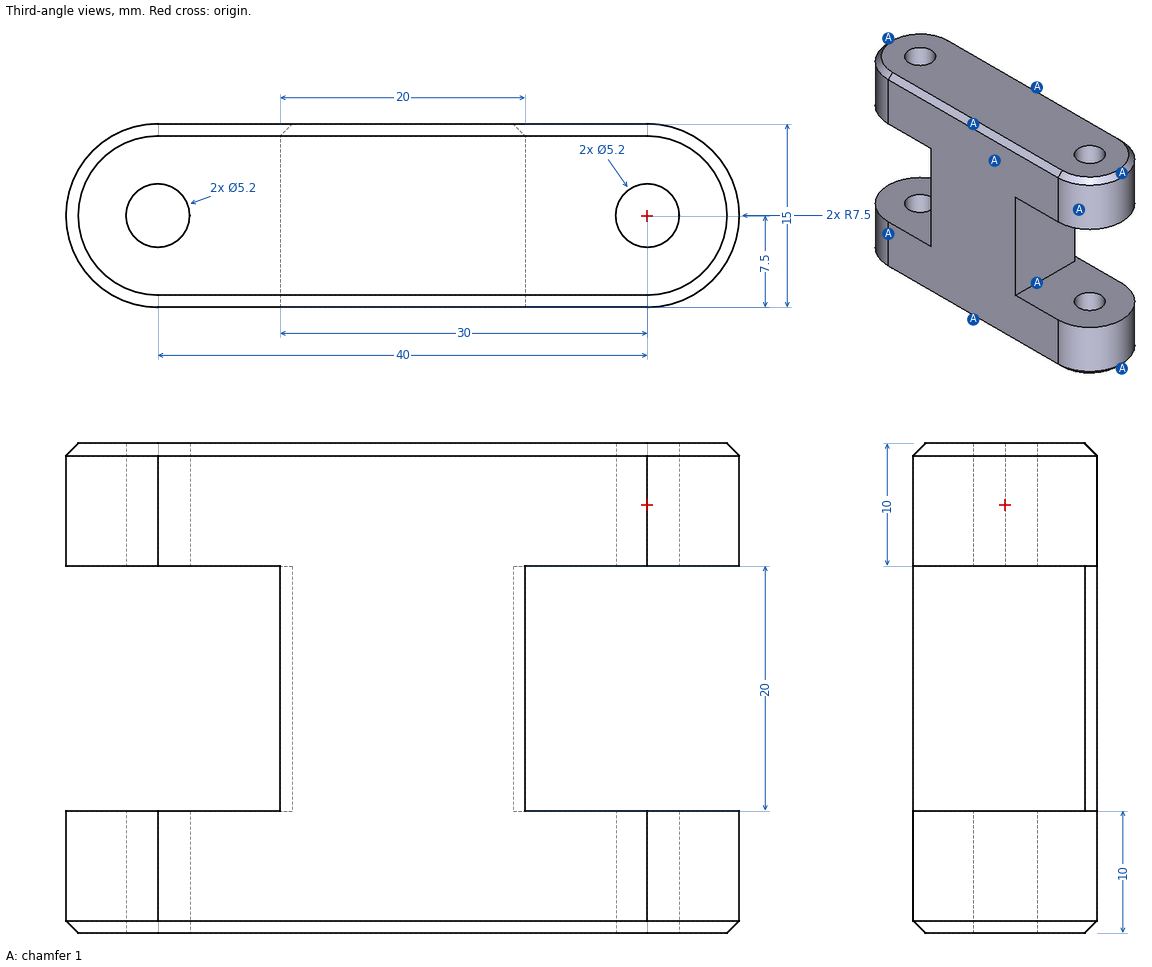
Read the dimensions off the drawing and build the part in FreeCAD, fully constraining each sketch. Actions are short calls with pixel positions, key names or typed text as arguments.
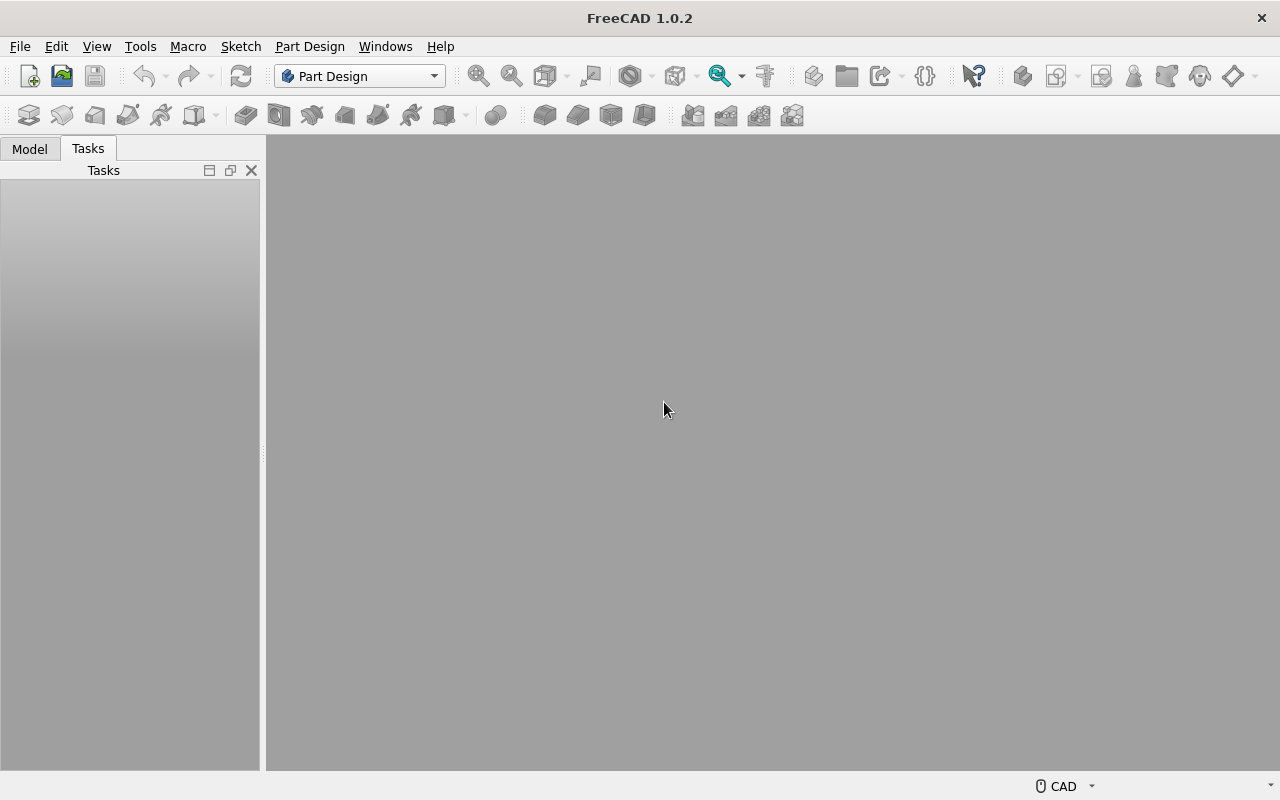
key(ctrl+n)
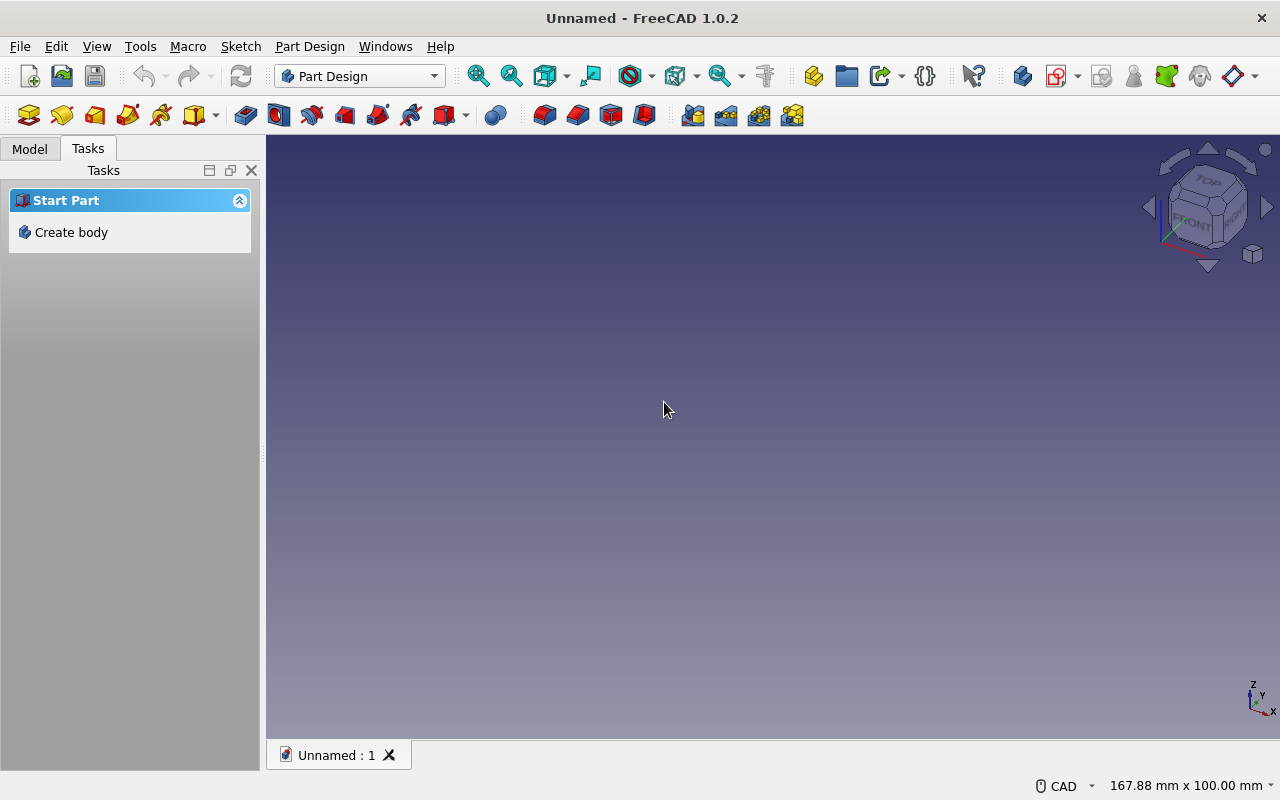
click(1056, 76)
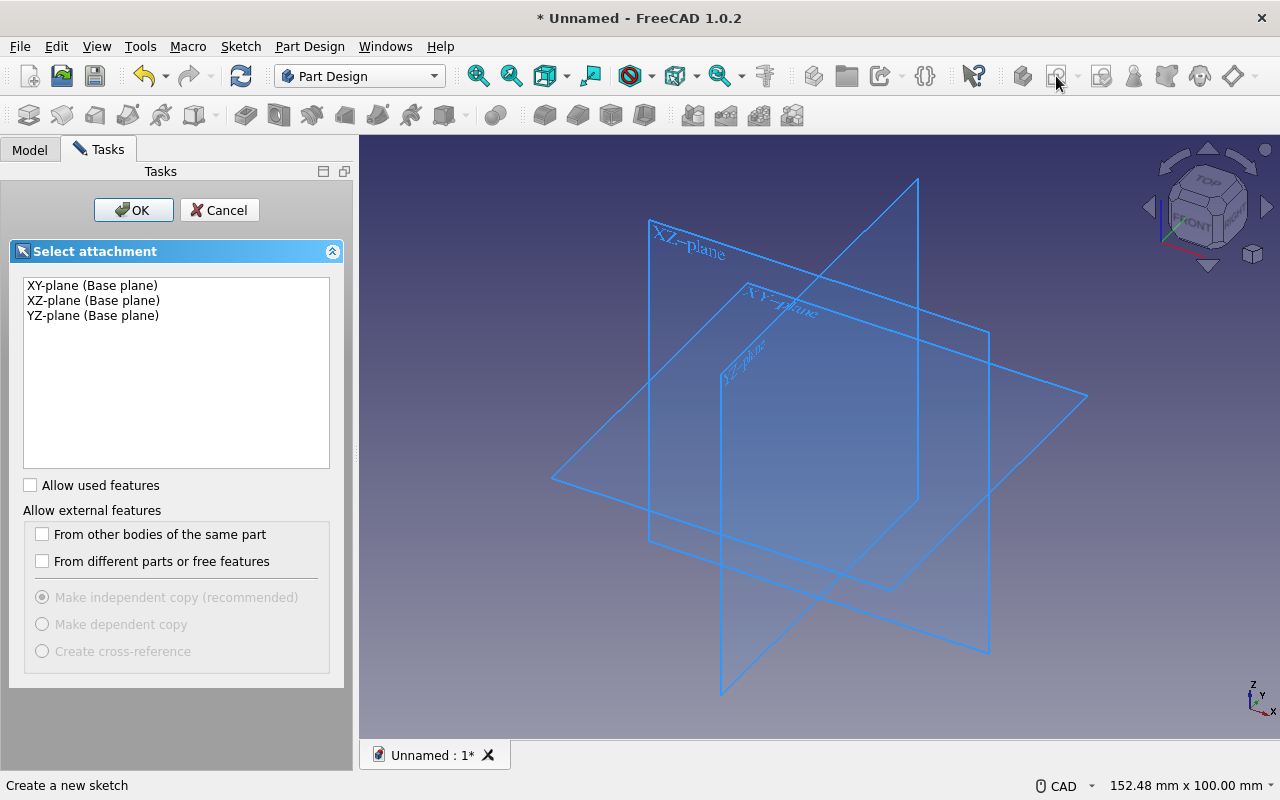
click(84, 286)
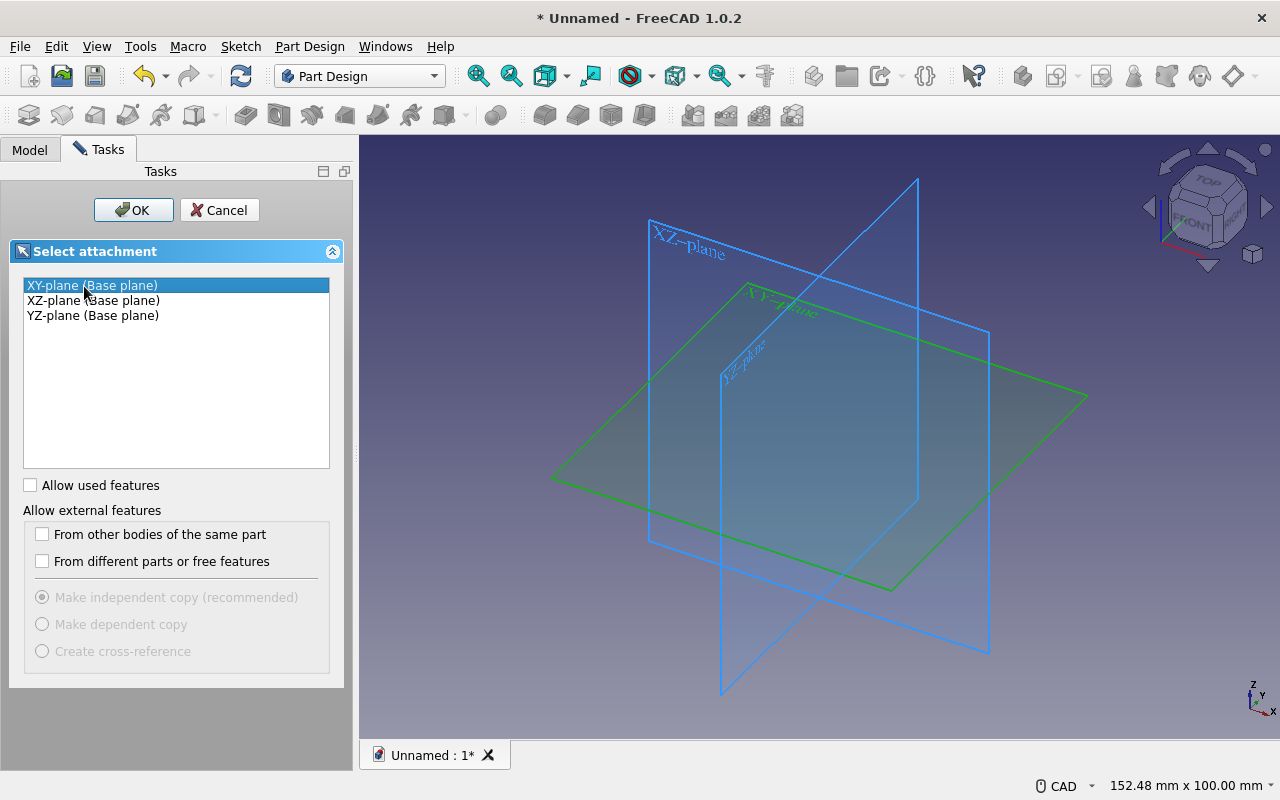
click(134, 210)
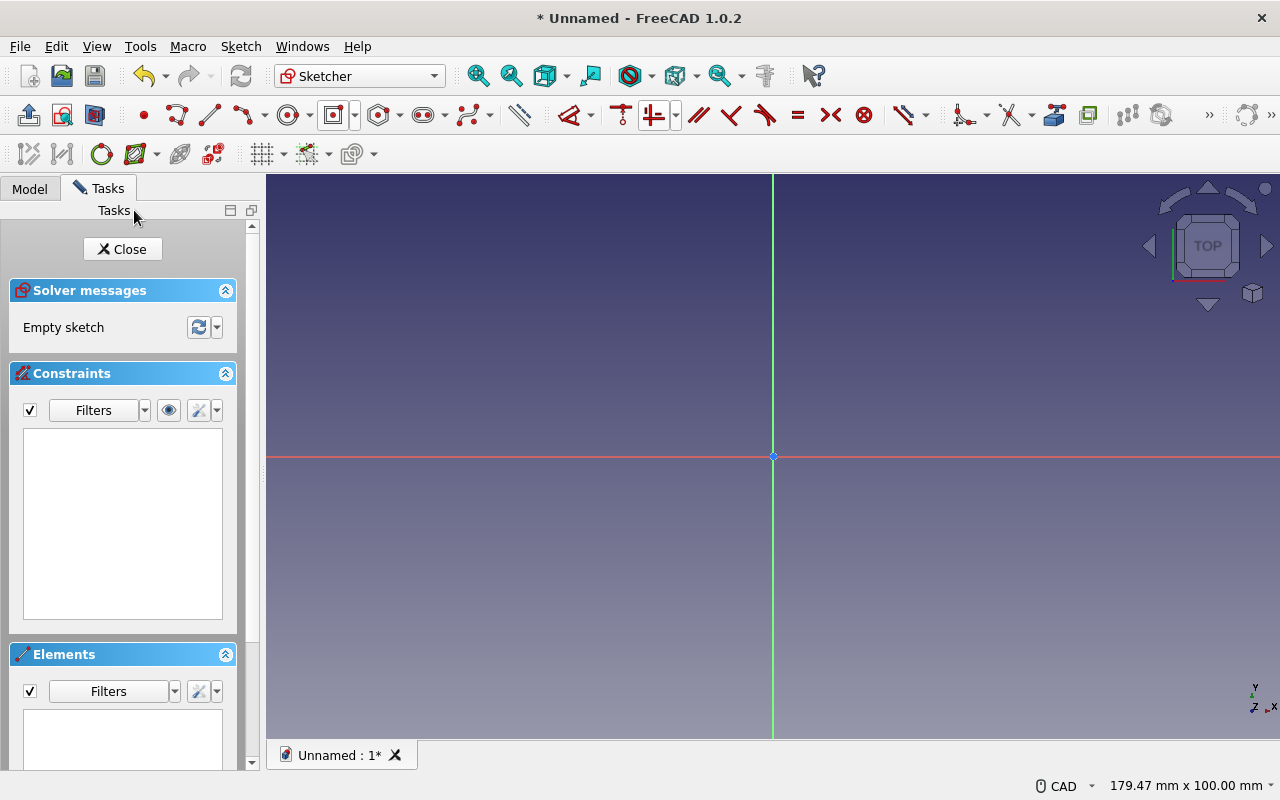
scroll(606, 456, up, 3)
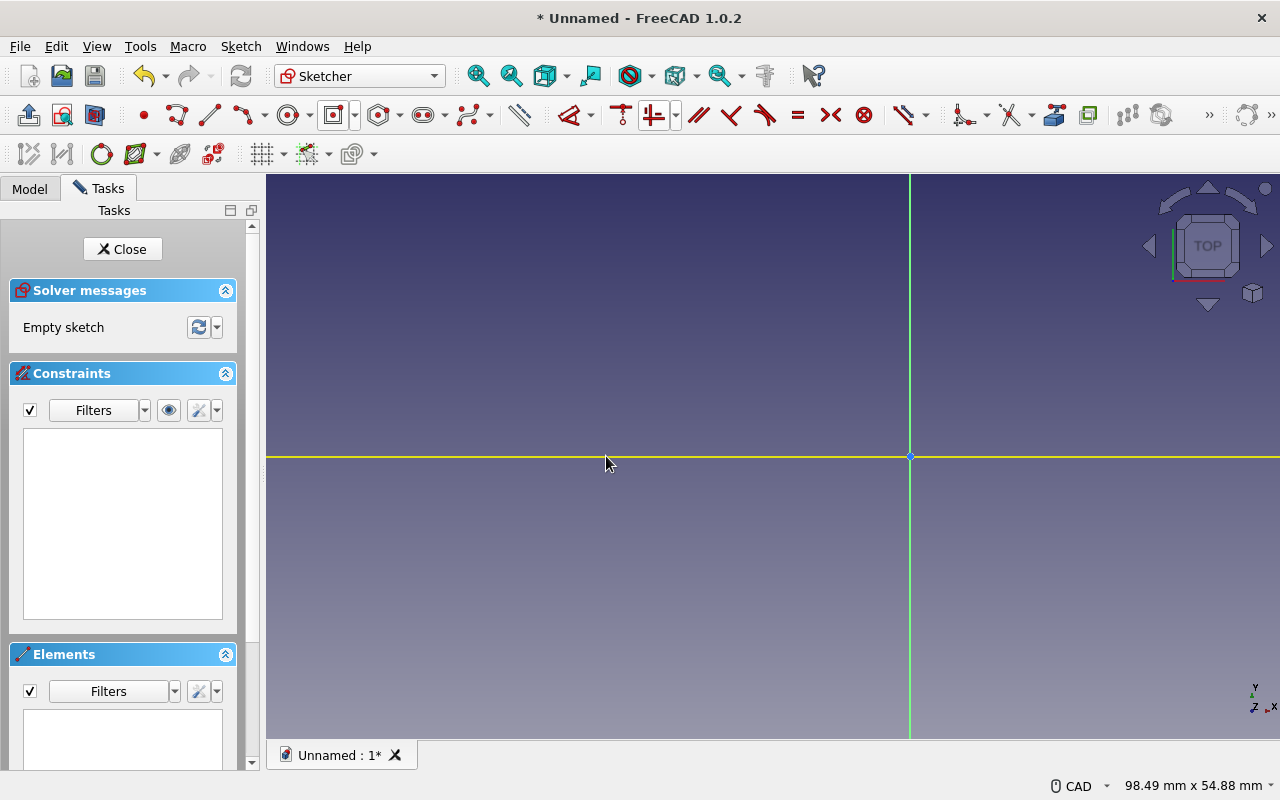
click(422, 116)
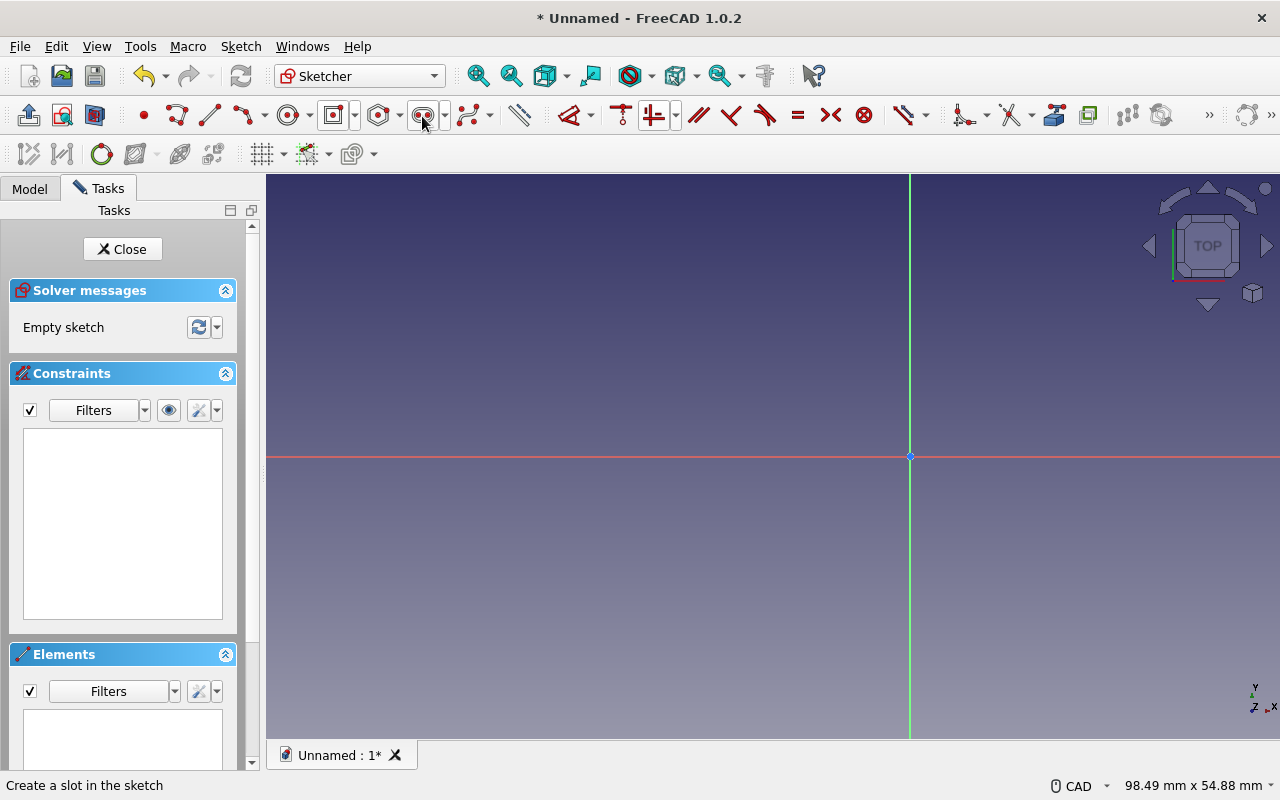
click(910, 456)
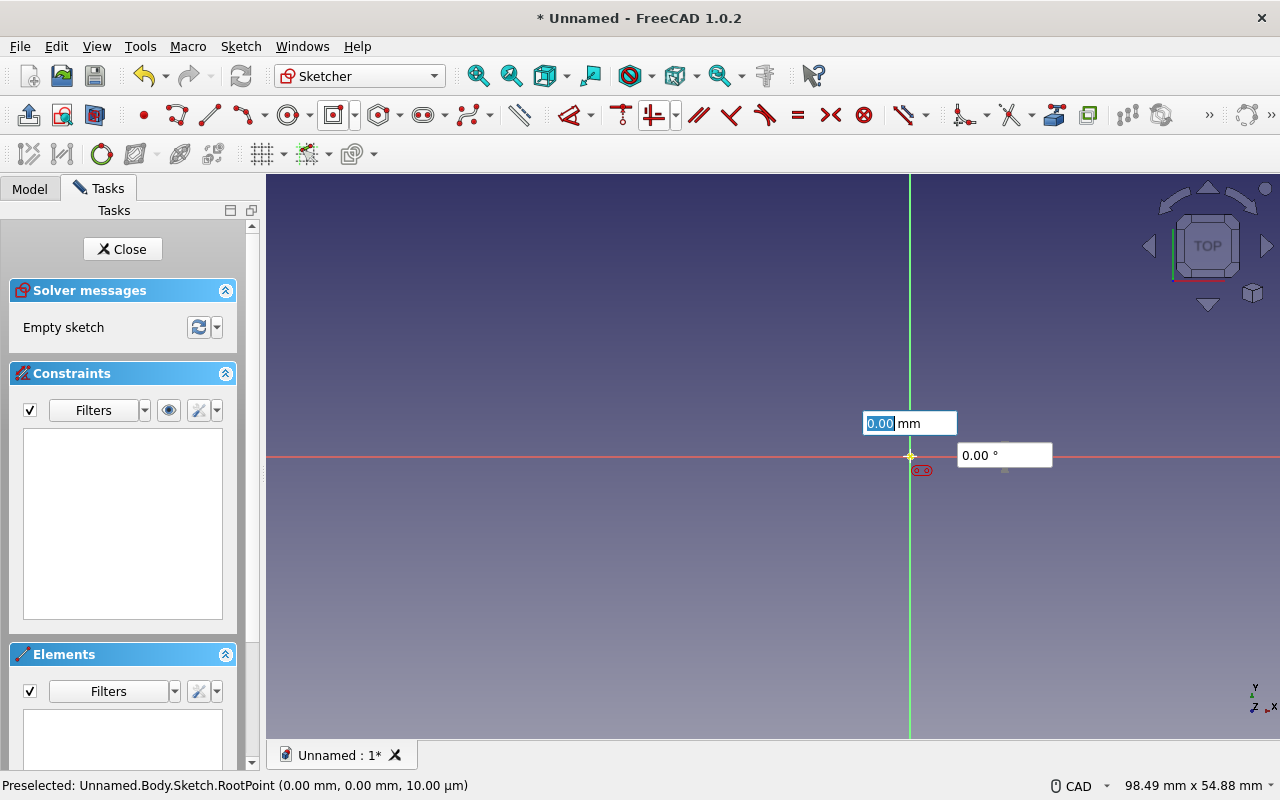
click(498, 448)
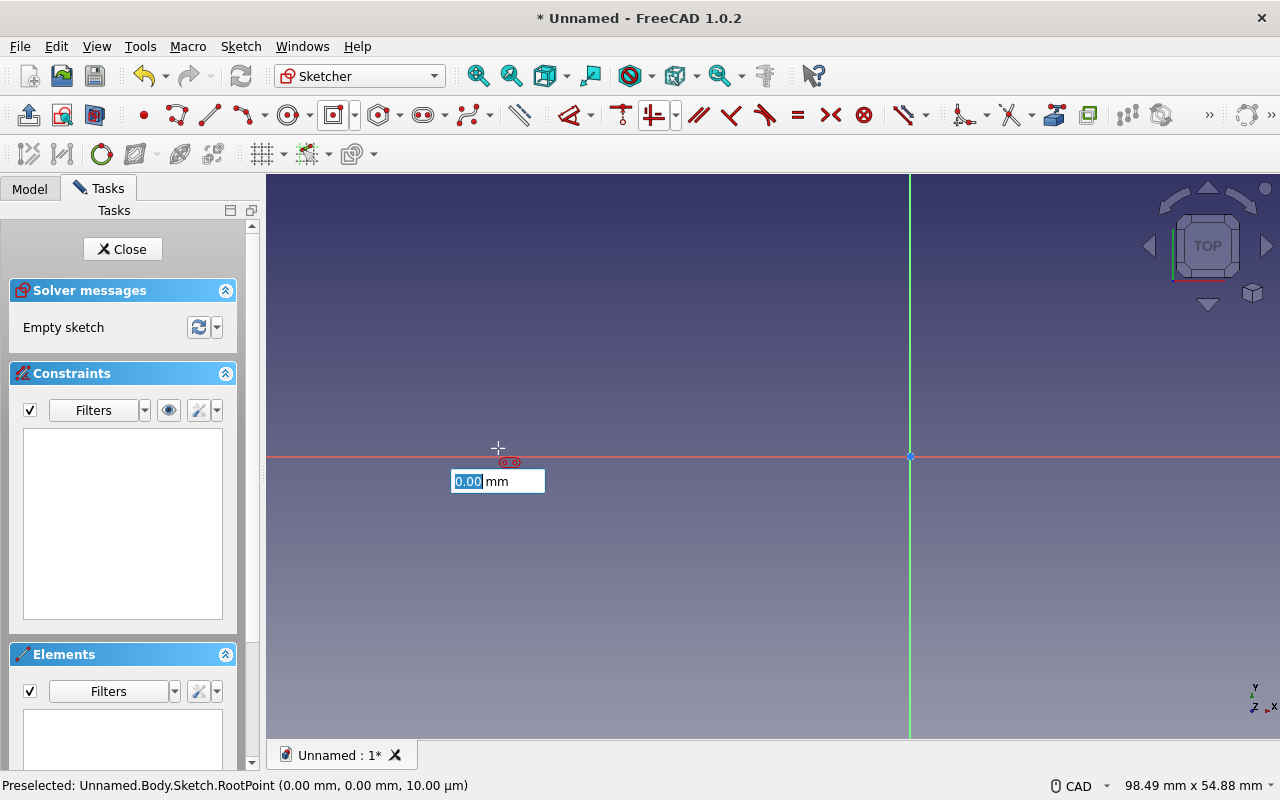
click(704, 534)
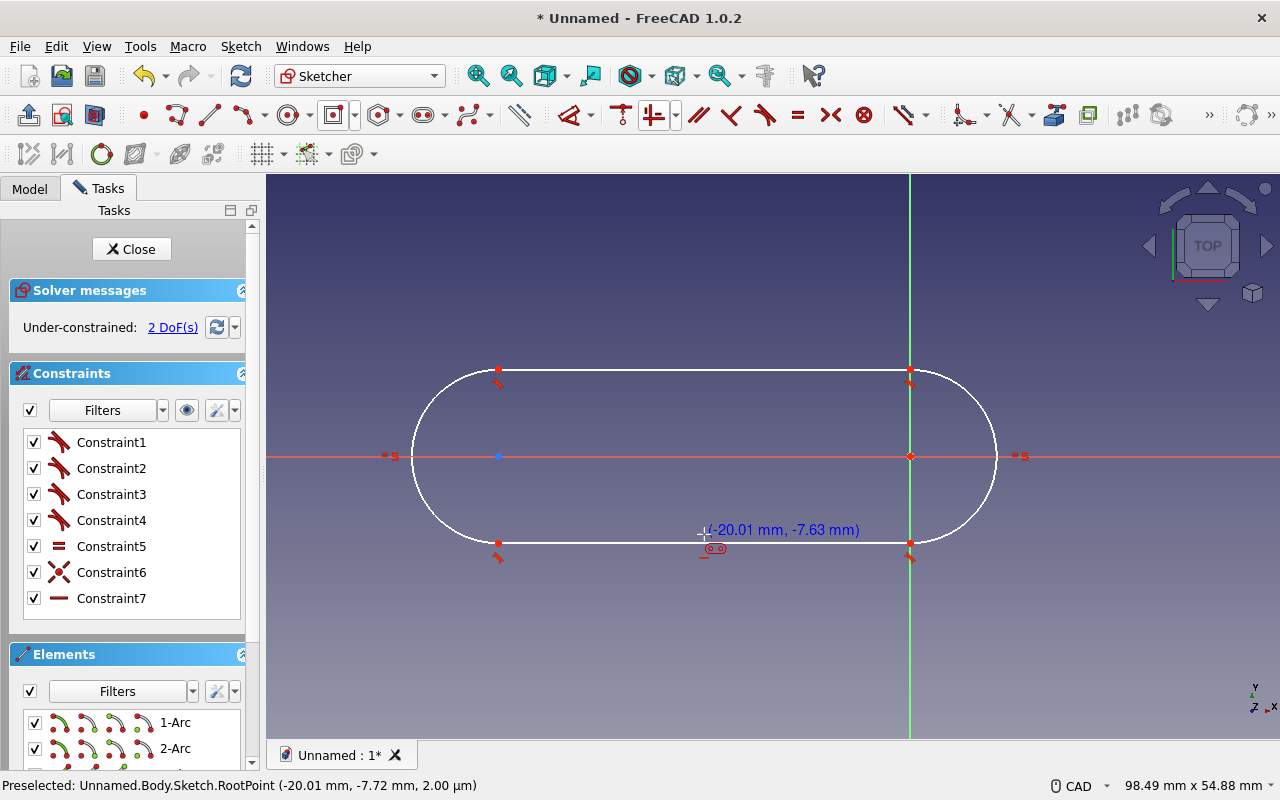
click(288, 116)